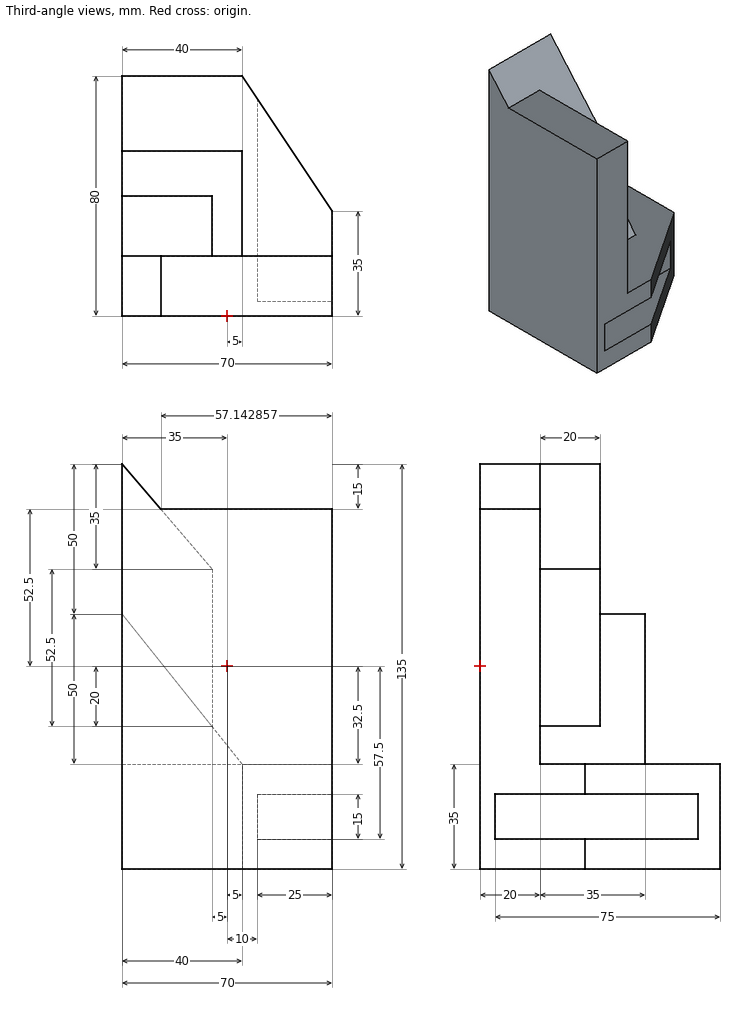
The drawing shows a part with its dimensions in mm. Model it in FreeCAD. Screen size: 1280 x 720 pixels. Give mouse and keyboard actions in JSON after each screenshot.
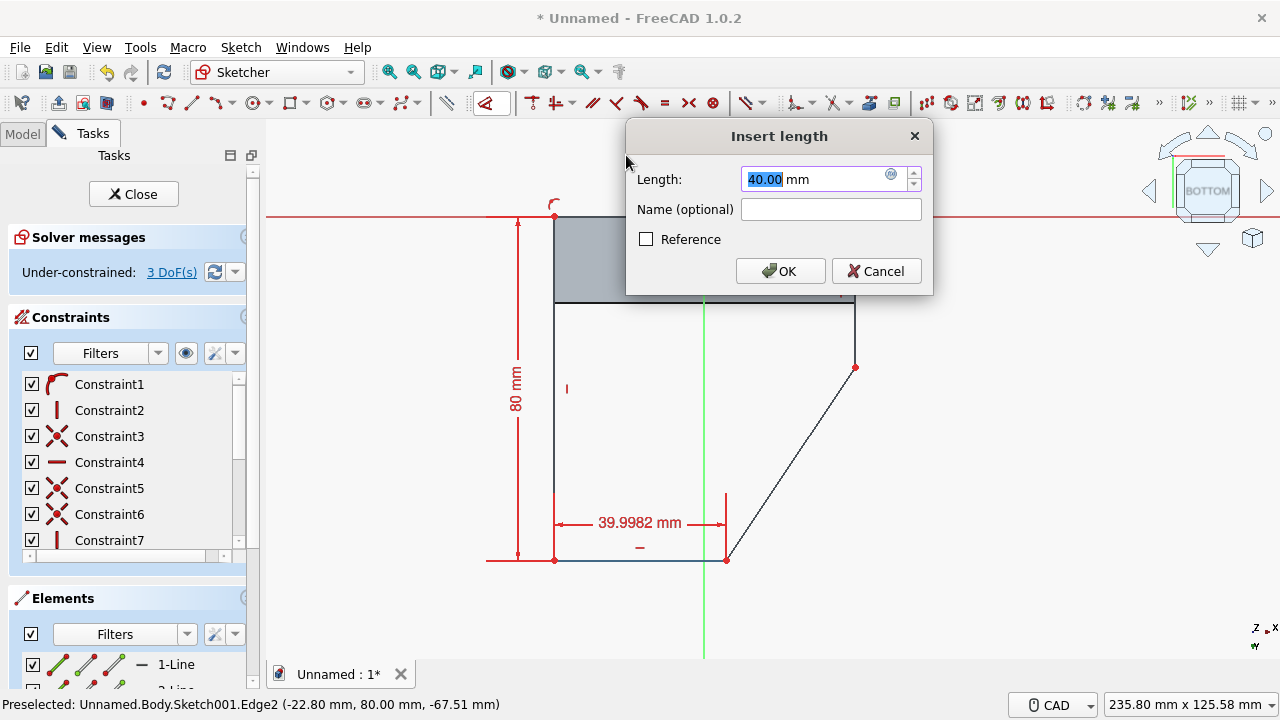
{"action": "type", "text": "40"}
{"action": "key", "text": "Return"}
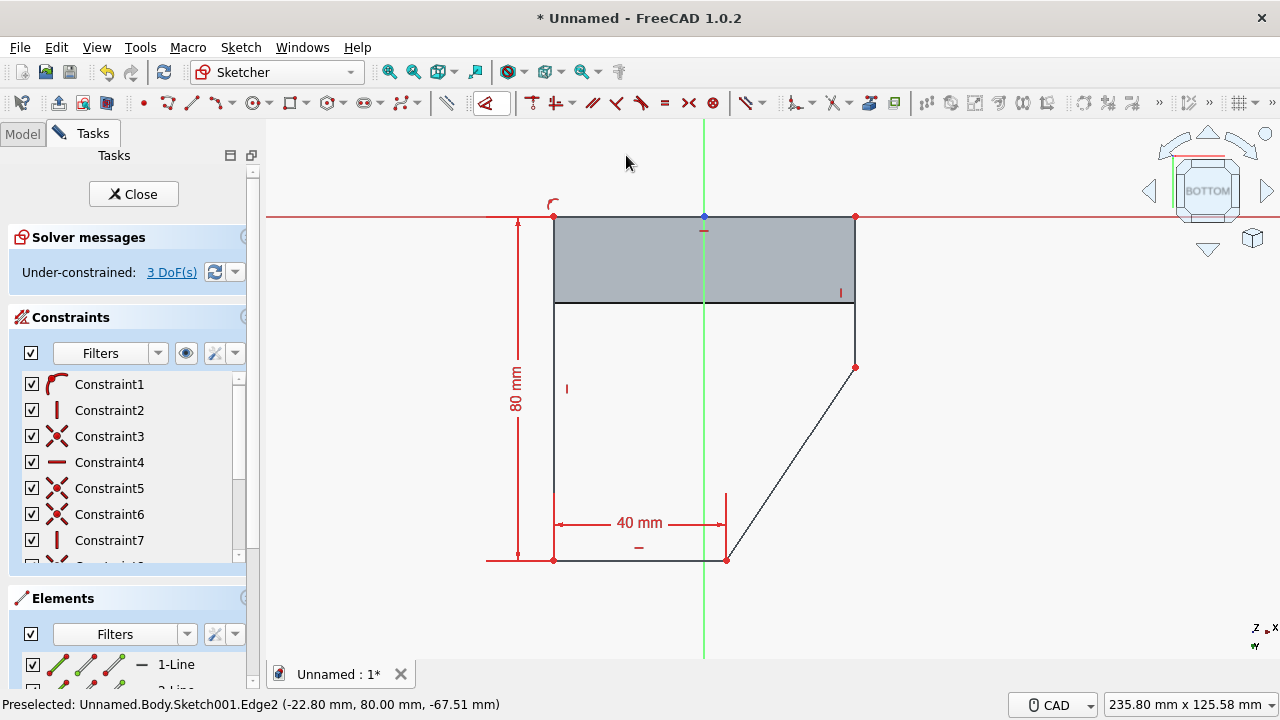
{"action": "left_click", "coordinate": [855, 323]}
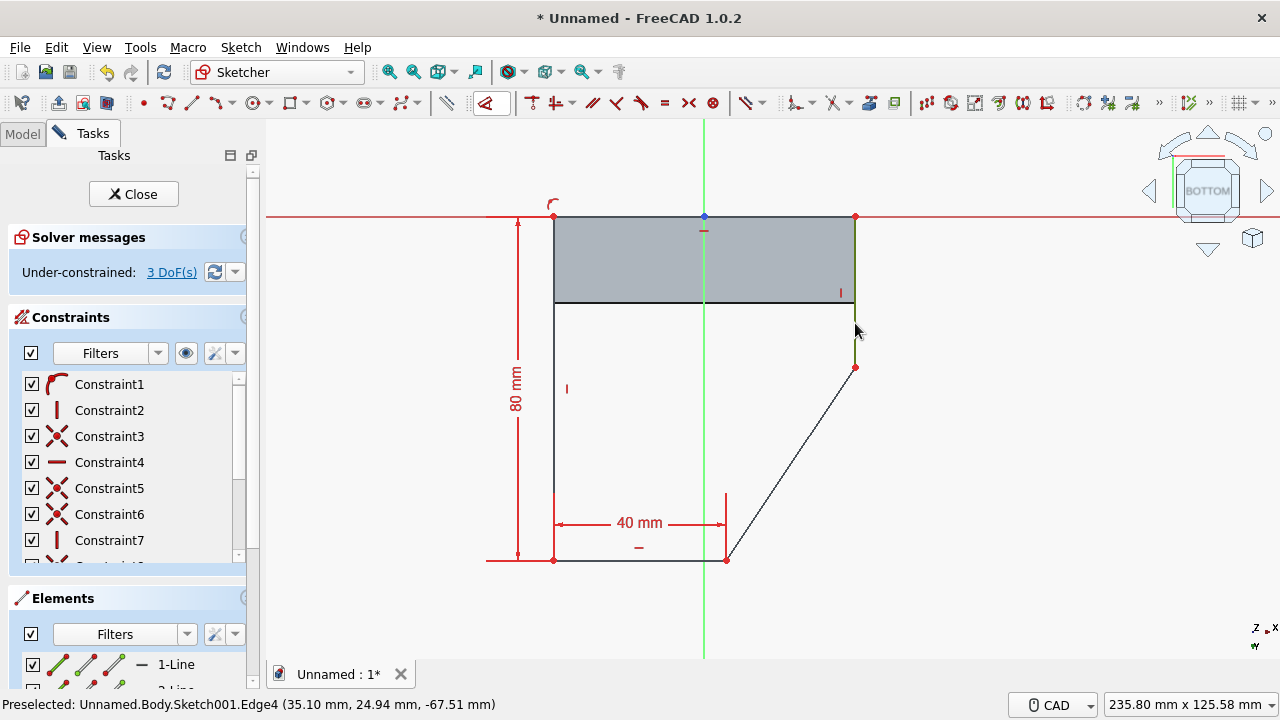
{"action": "left_click", "coordinate": [504, 104]}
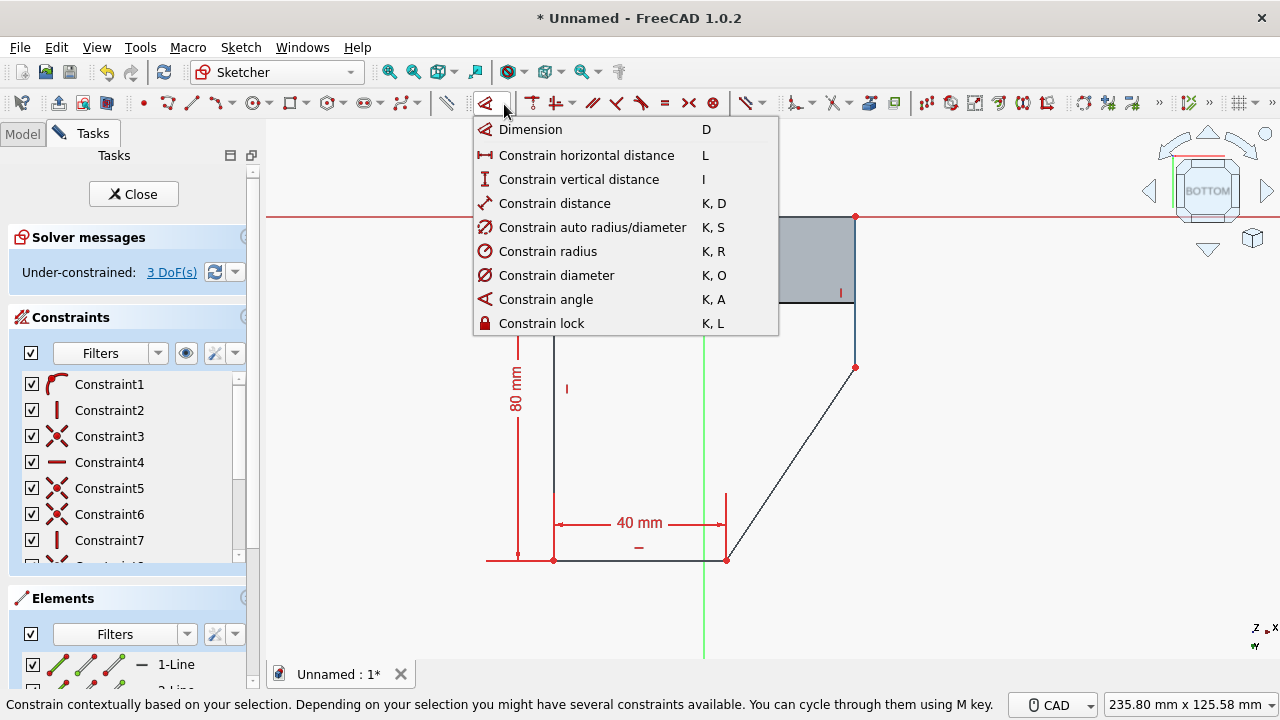
{"action": "left_click", "coordinate": [626, 179]}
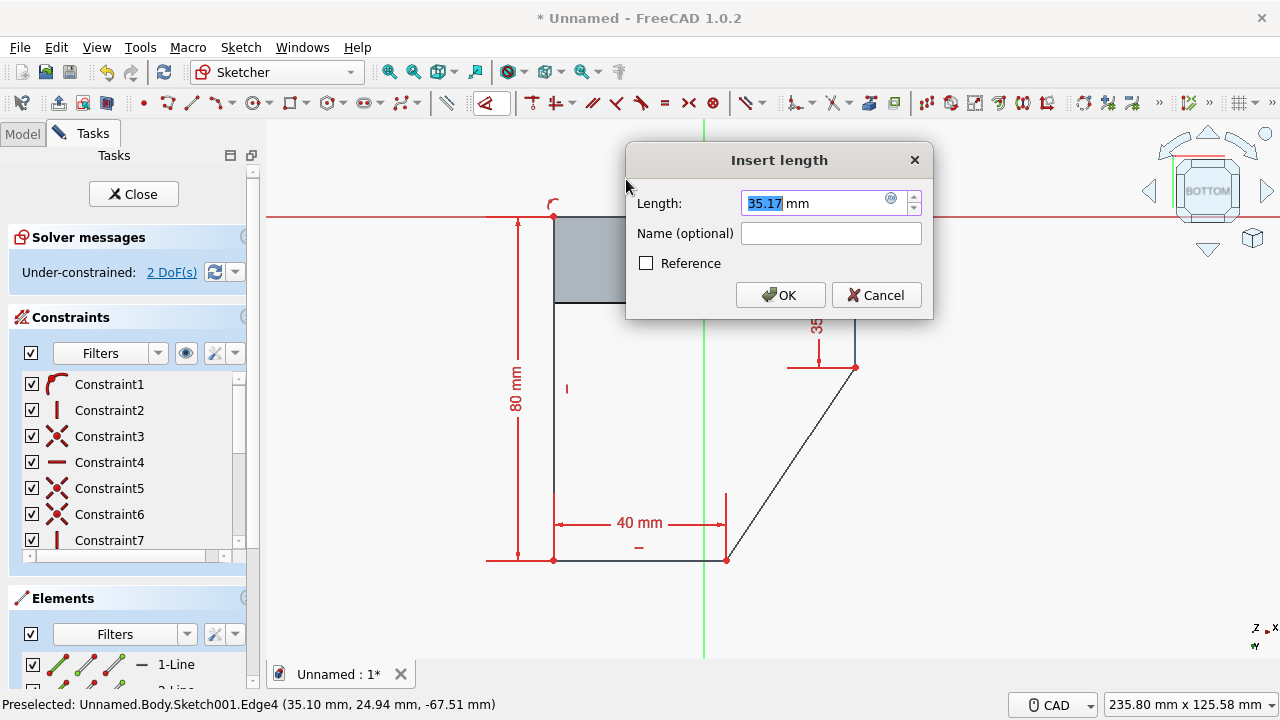
{"action": "type", "text": "35"}
{"action": "key", "text": "Return"}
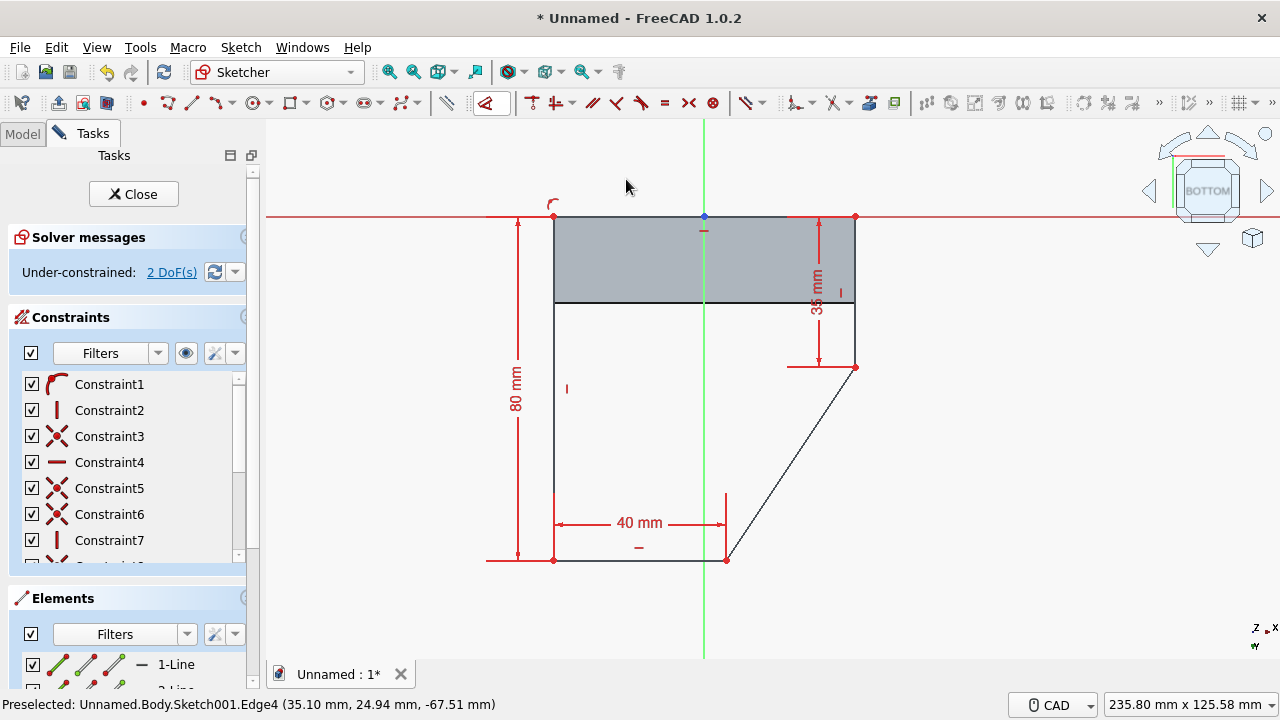
{"action": "left_click", "coordinate": [765, 217]}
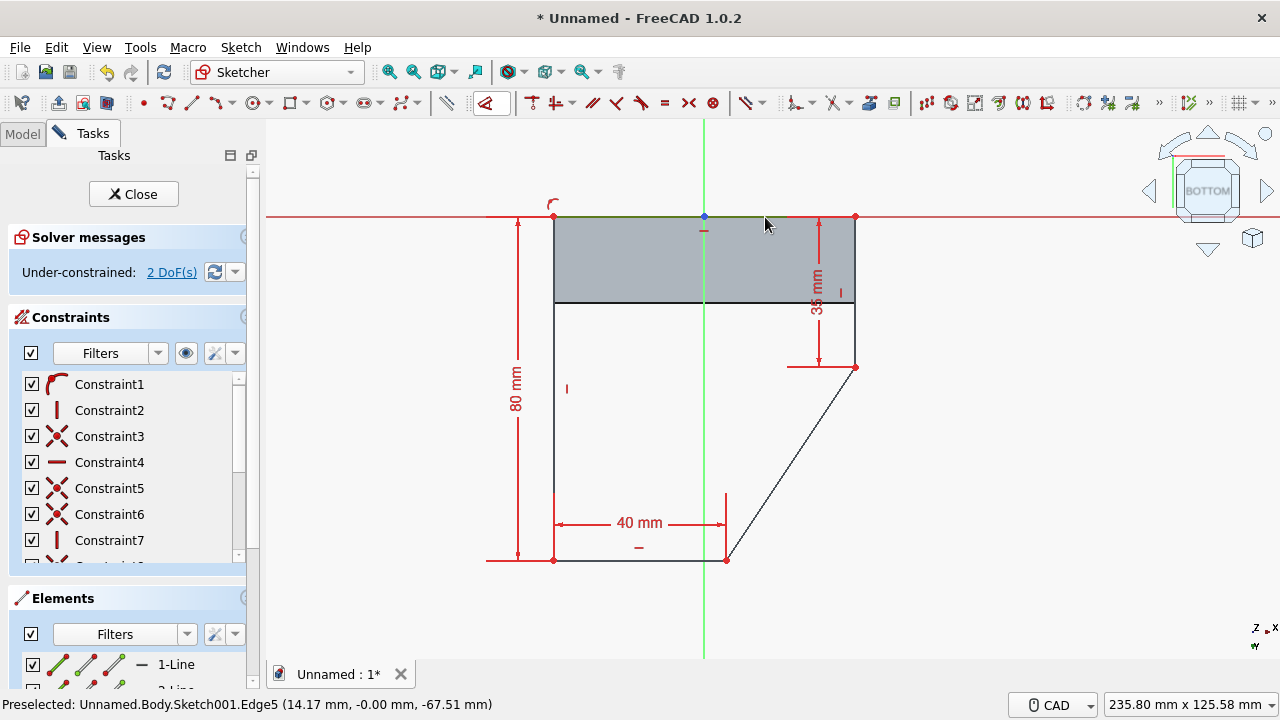
{"action": "left_click", "coordinate": [504, 104]}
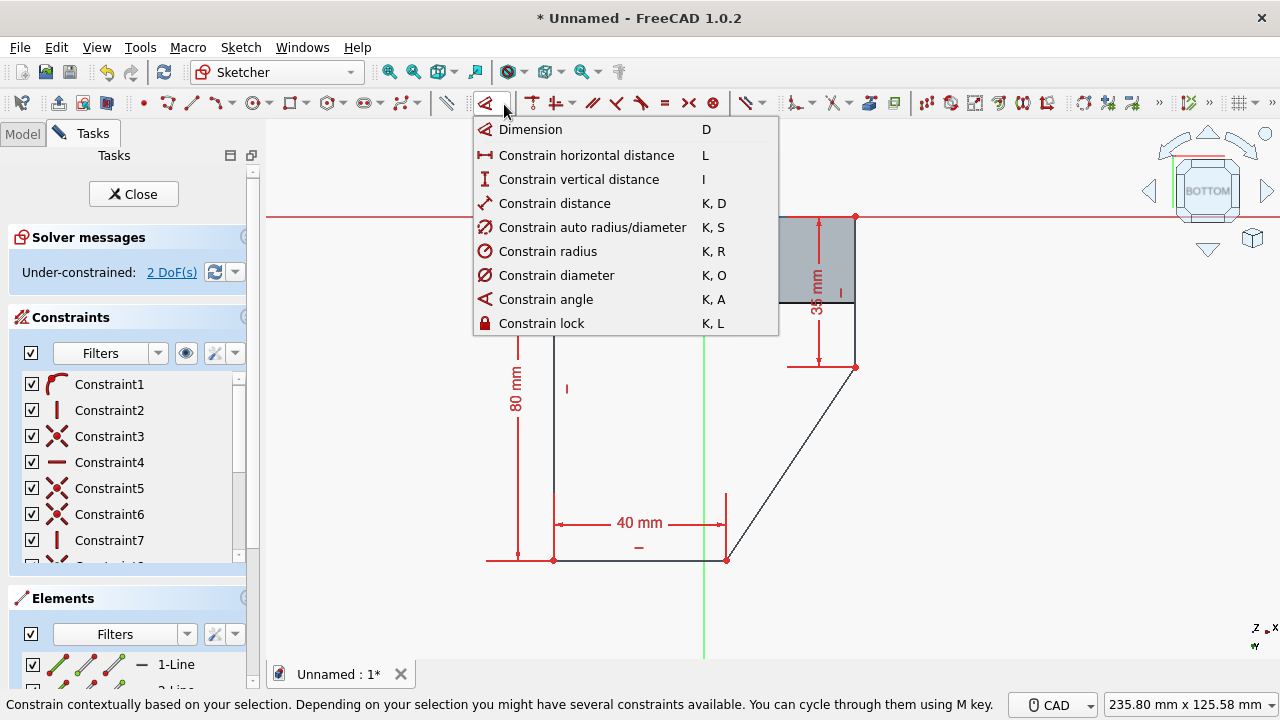
{"action": "left_click", "coordinate": [626, 155]}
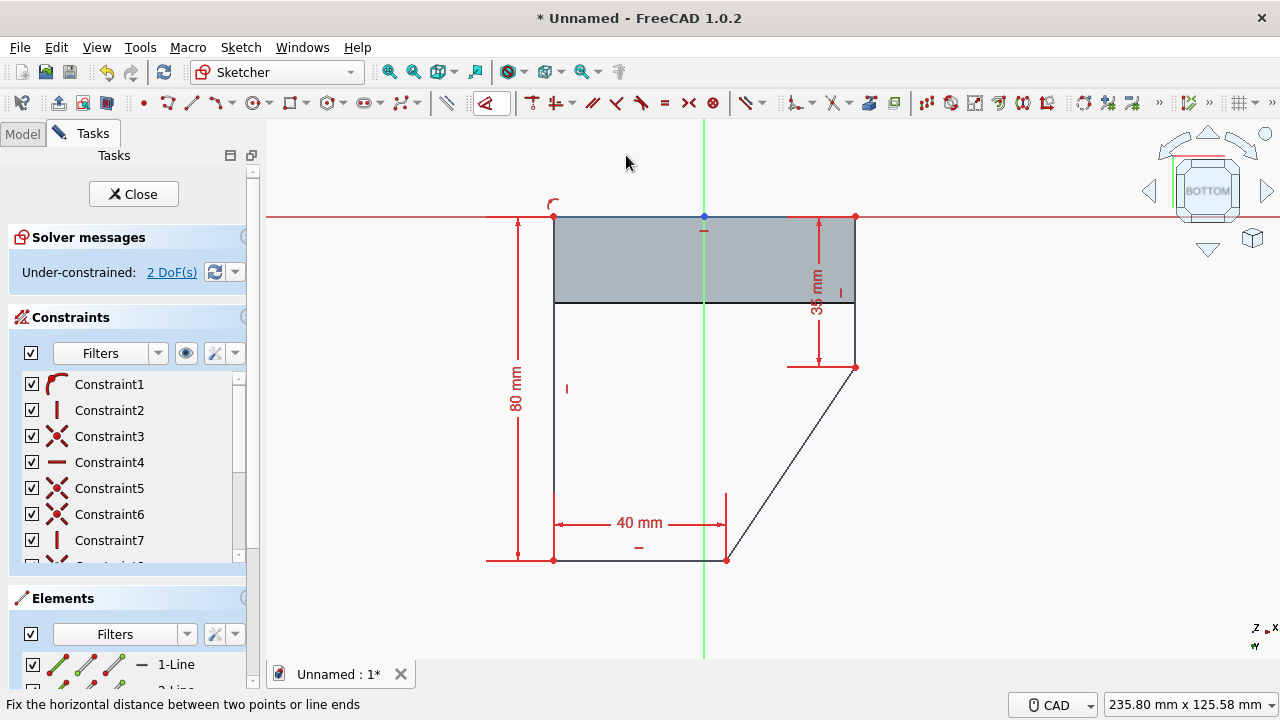
{"action": "type", "text": "70"}
{"action": "key", "text": "Return"}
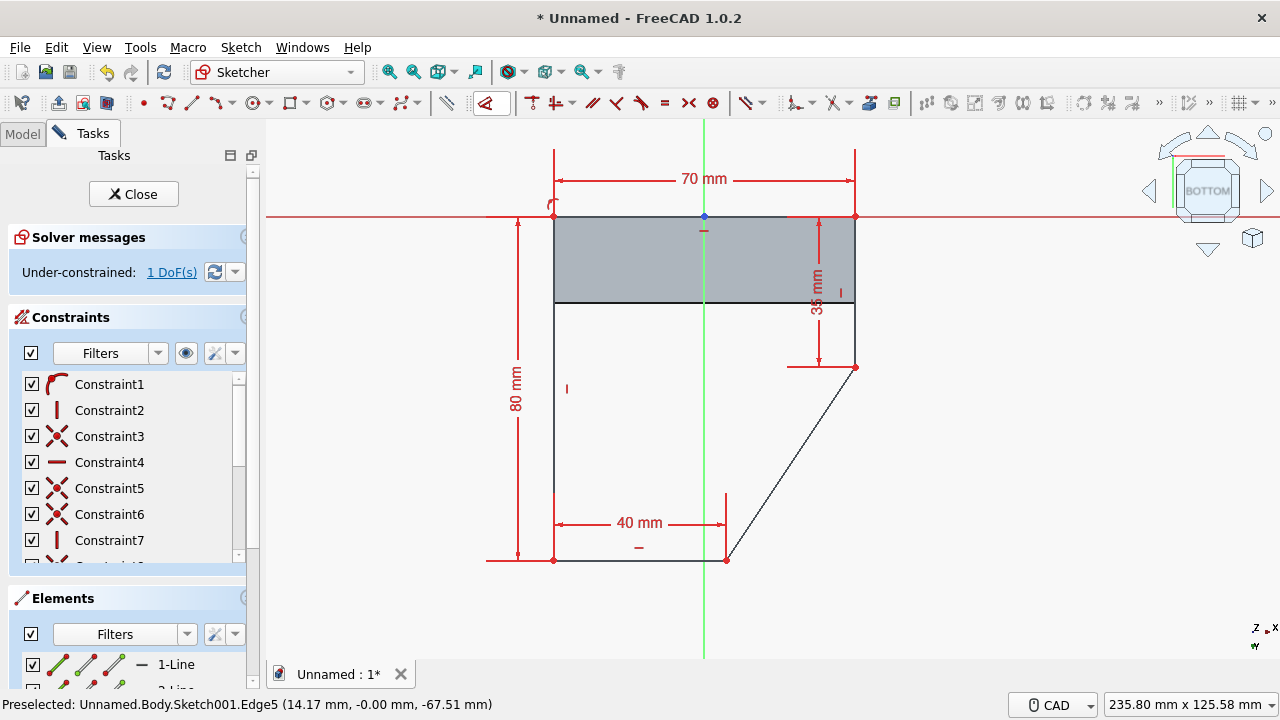
{"action": "scroll", "coordinate": [726, 561], "scroll_direction": "up", "scroll_amount": 4}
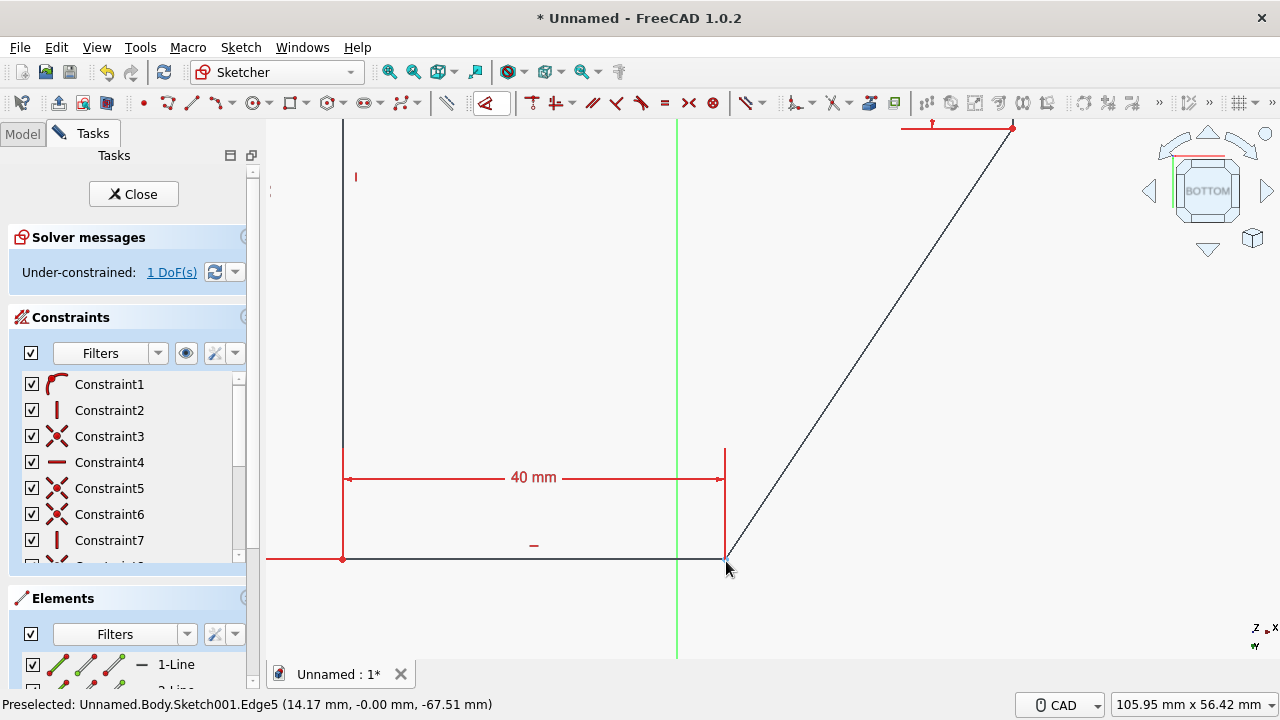
{"action": "left_click", "coordinate": [725, 559]}